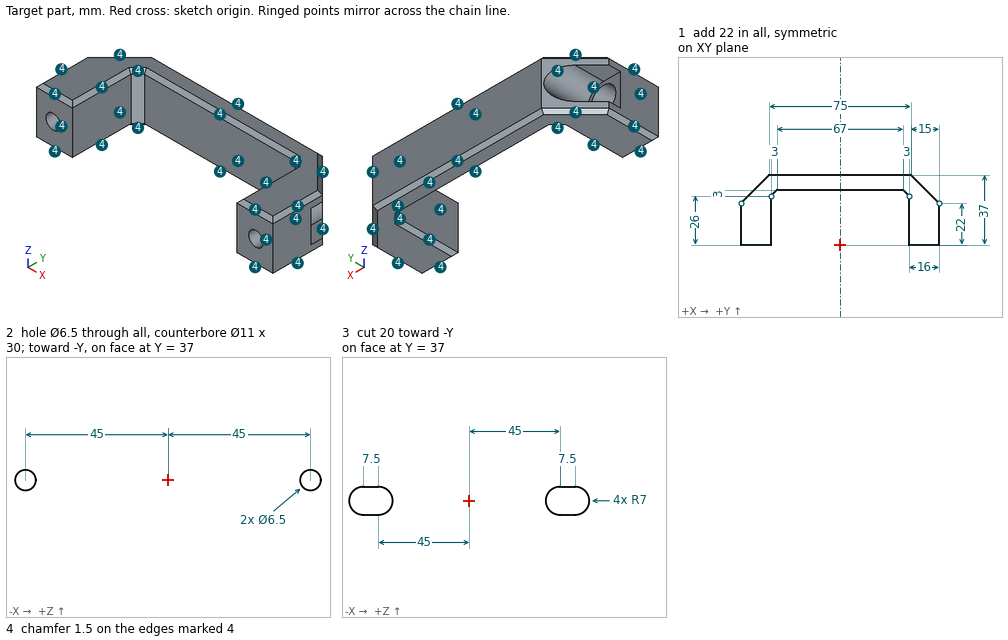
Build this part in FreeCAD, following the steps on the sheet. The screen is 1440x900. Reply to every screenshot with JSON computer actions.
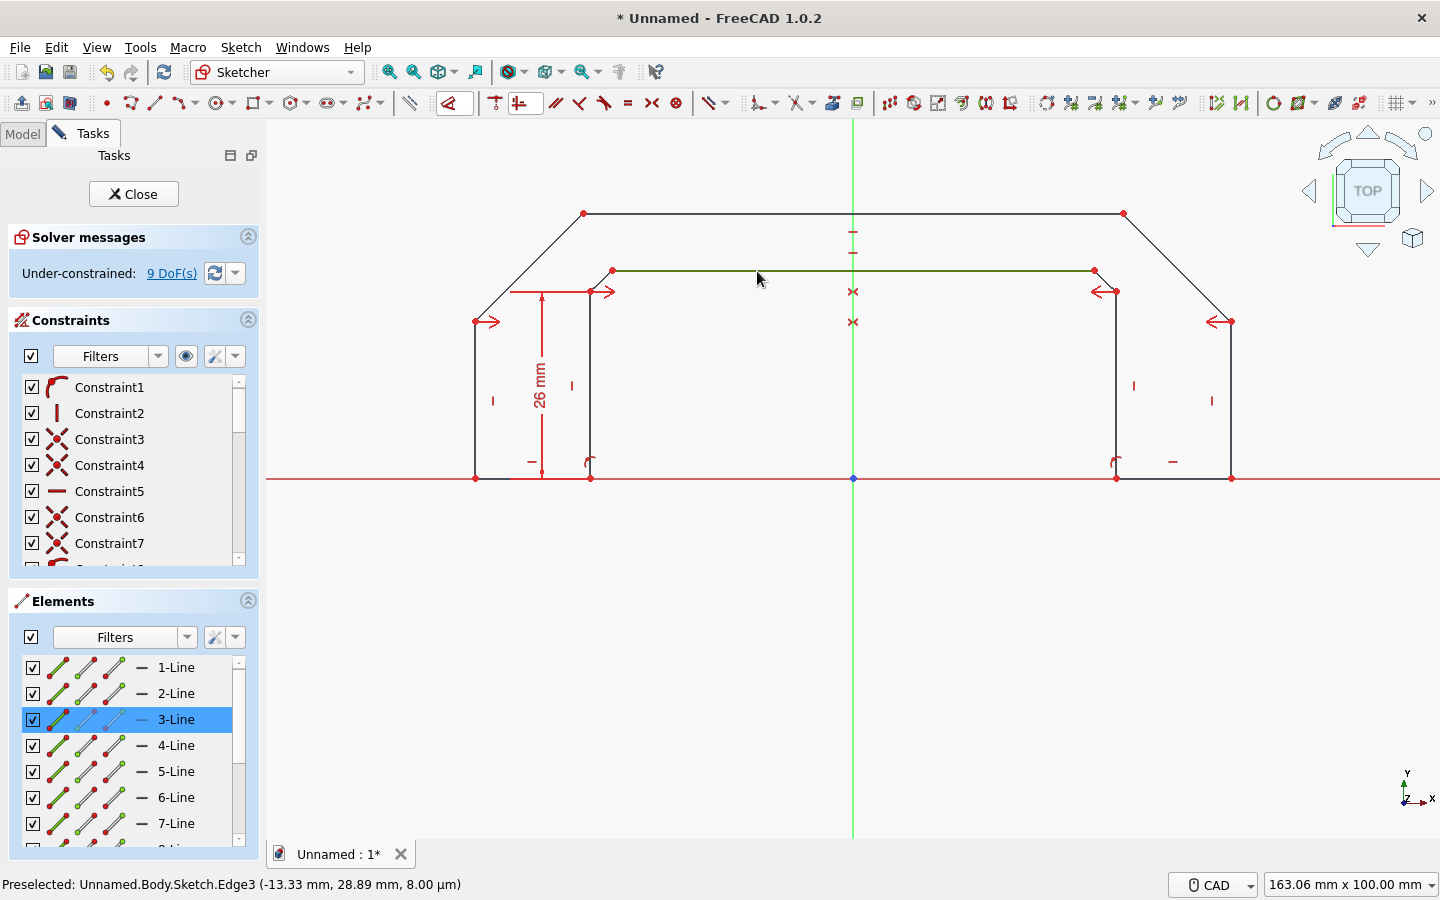
{"action": "left_click", "coordinate": [468, 104]}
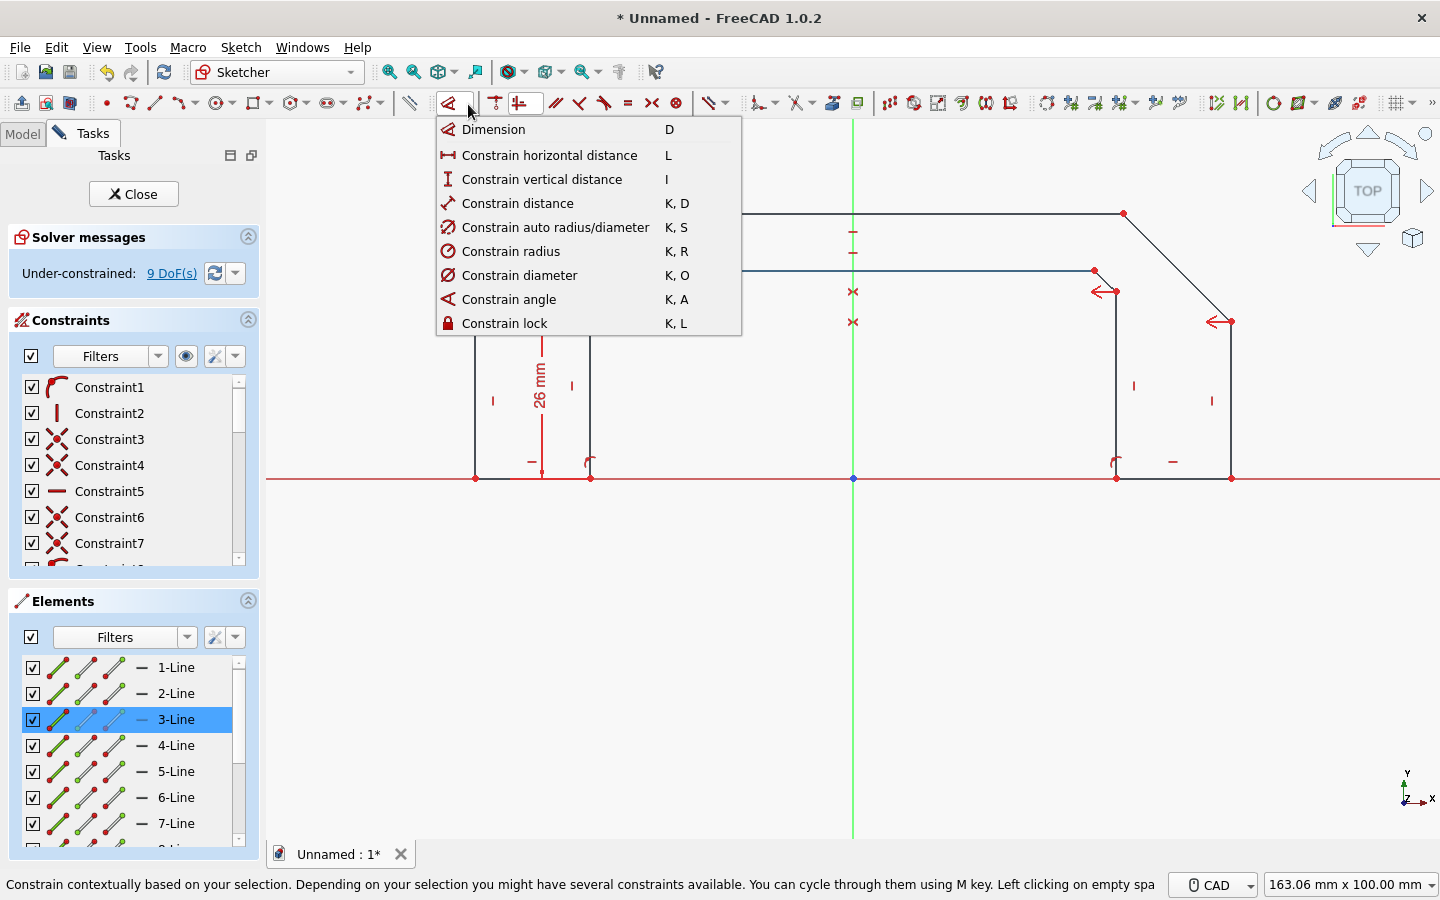
{"action": "left_click", "coordinate": [589, 155]}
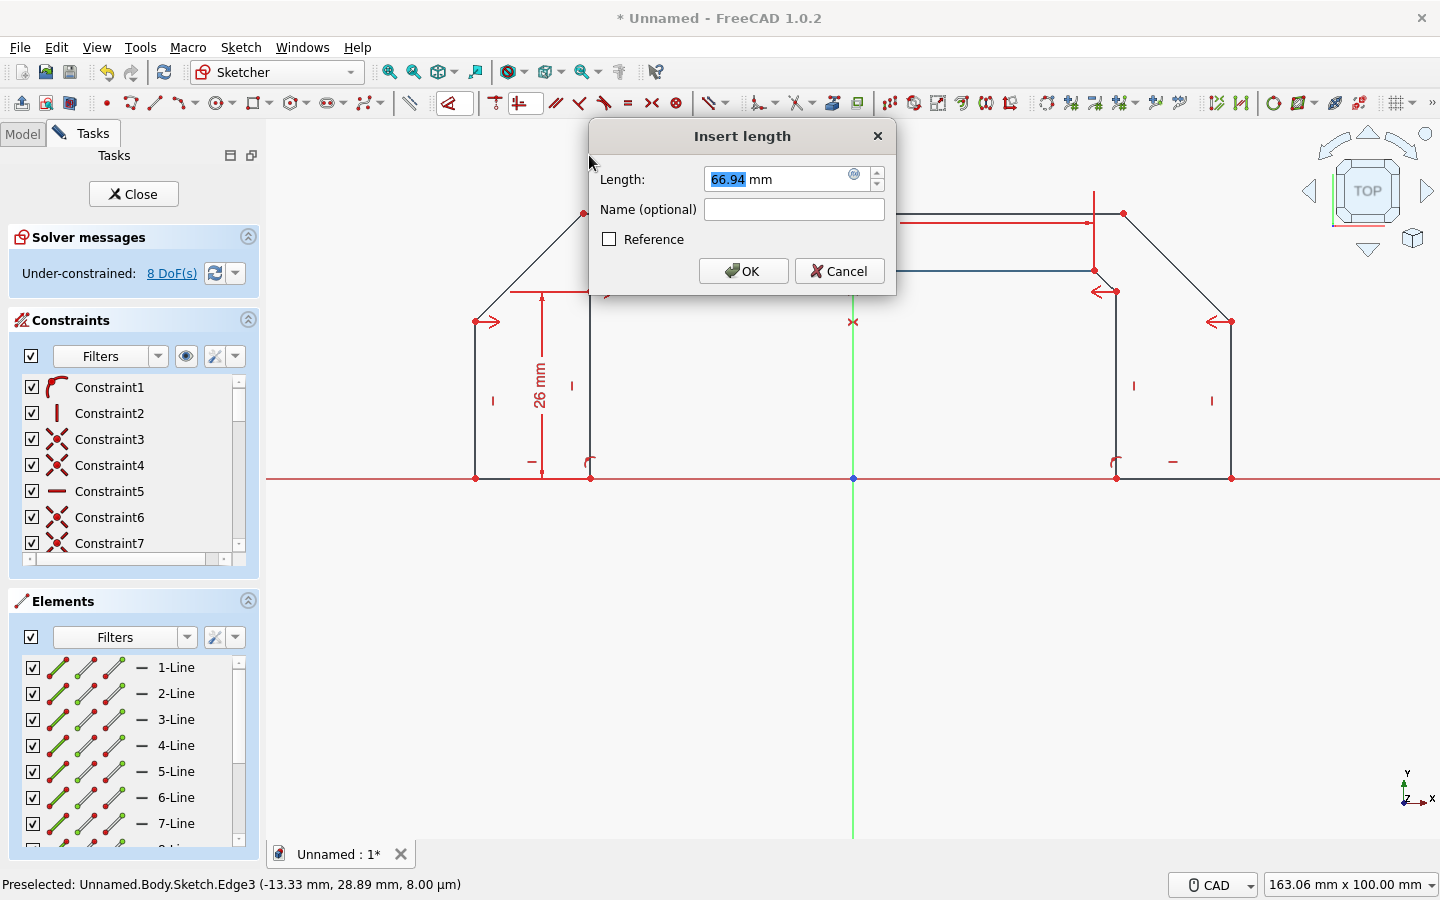
{"action": "type", "text": "67"}
{"action": "key", "text": "Return"}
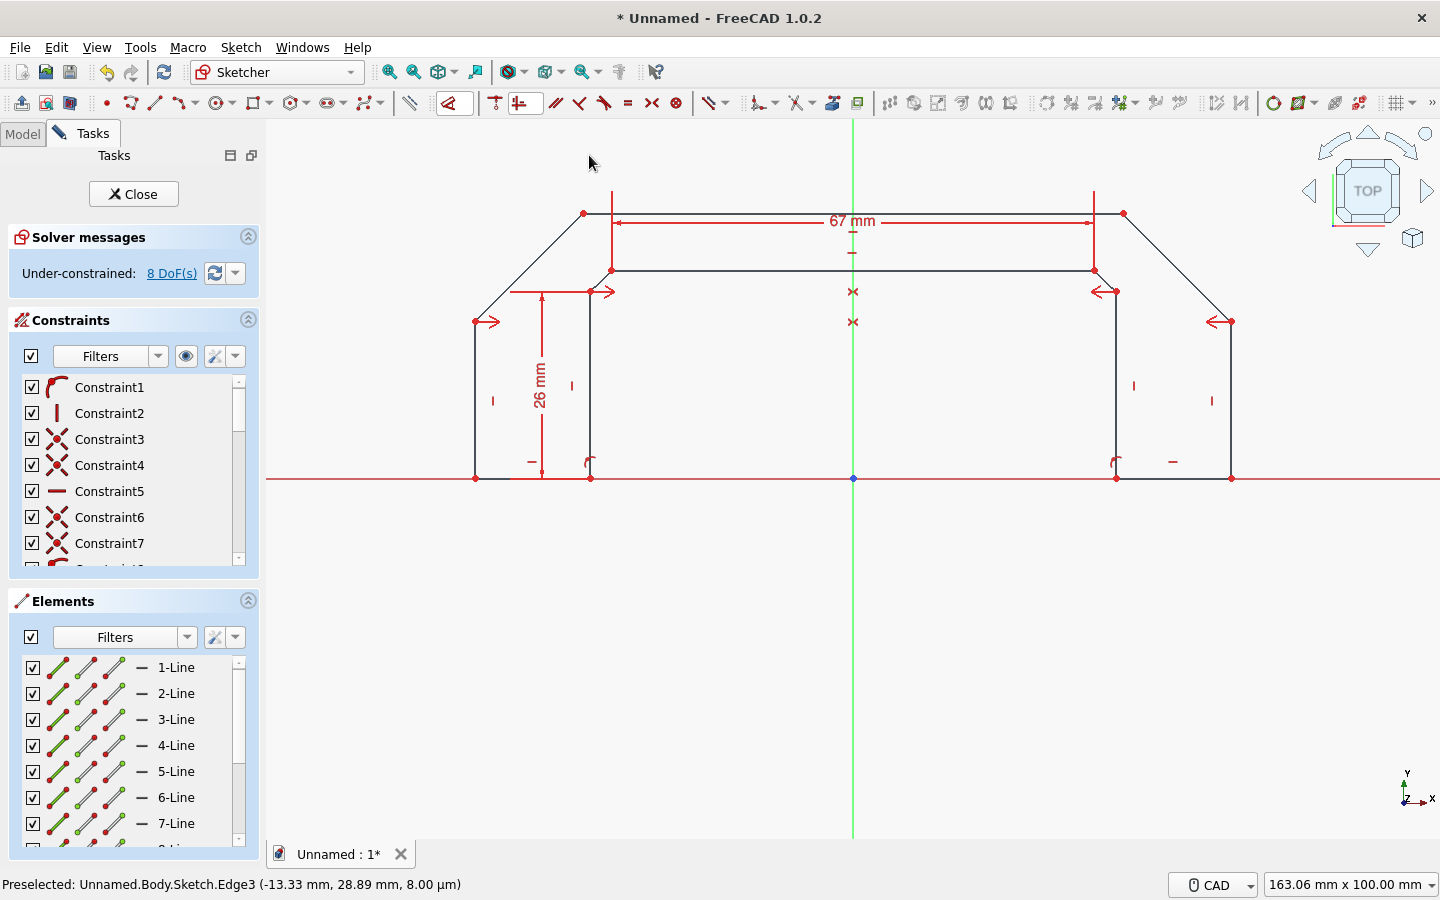
{"action": "left_click", "coordinate": [1150, 479]}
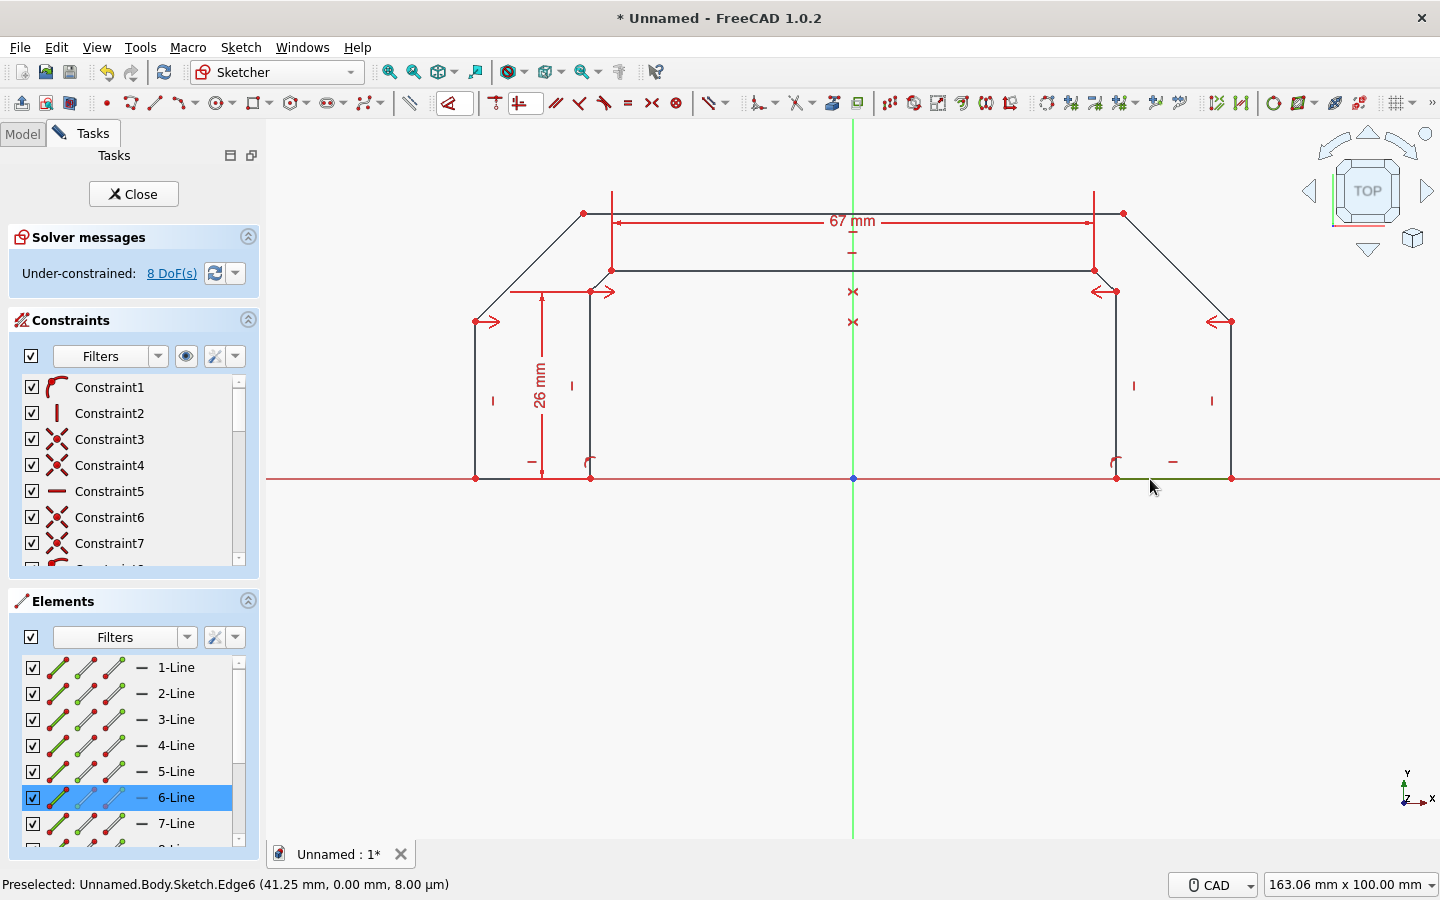
{"action": "left_click", "coordinate": [468, 104]}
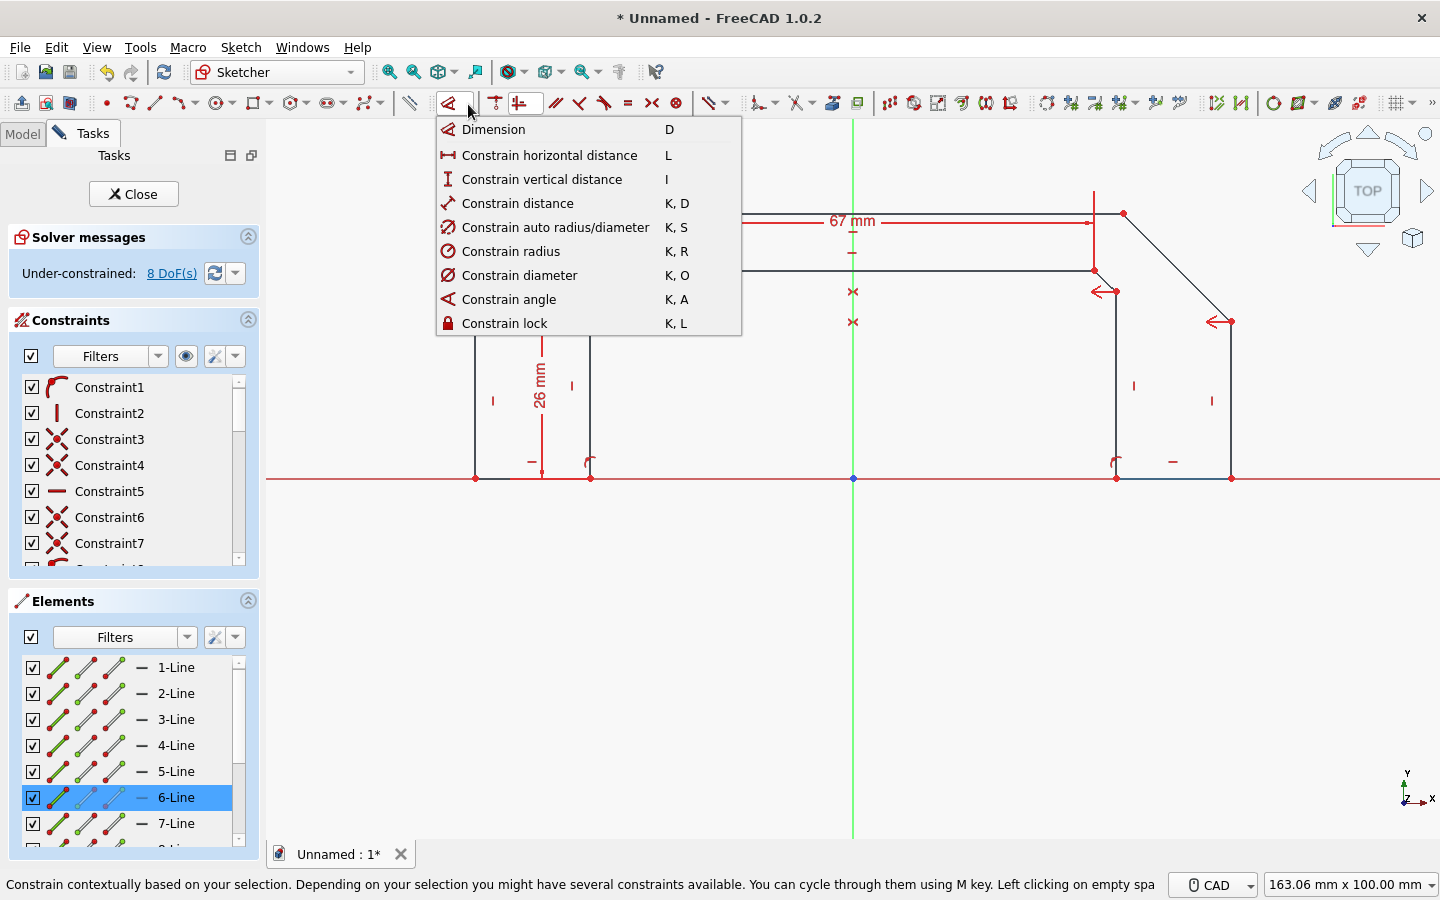
{"action": "left_click", "coordinate": [589, 155]}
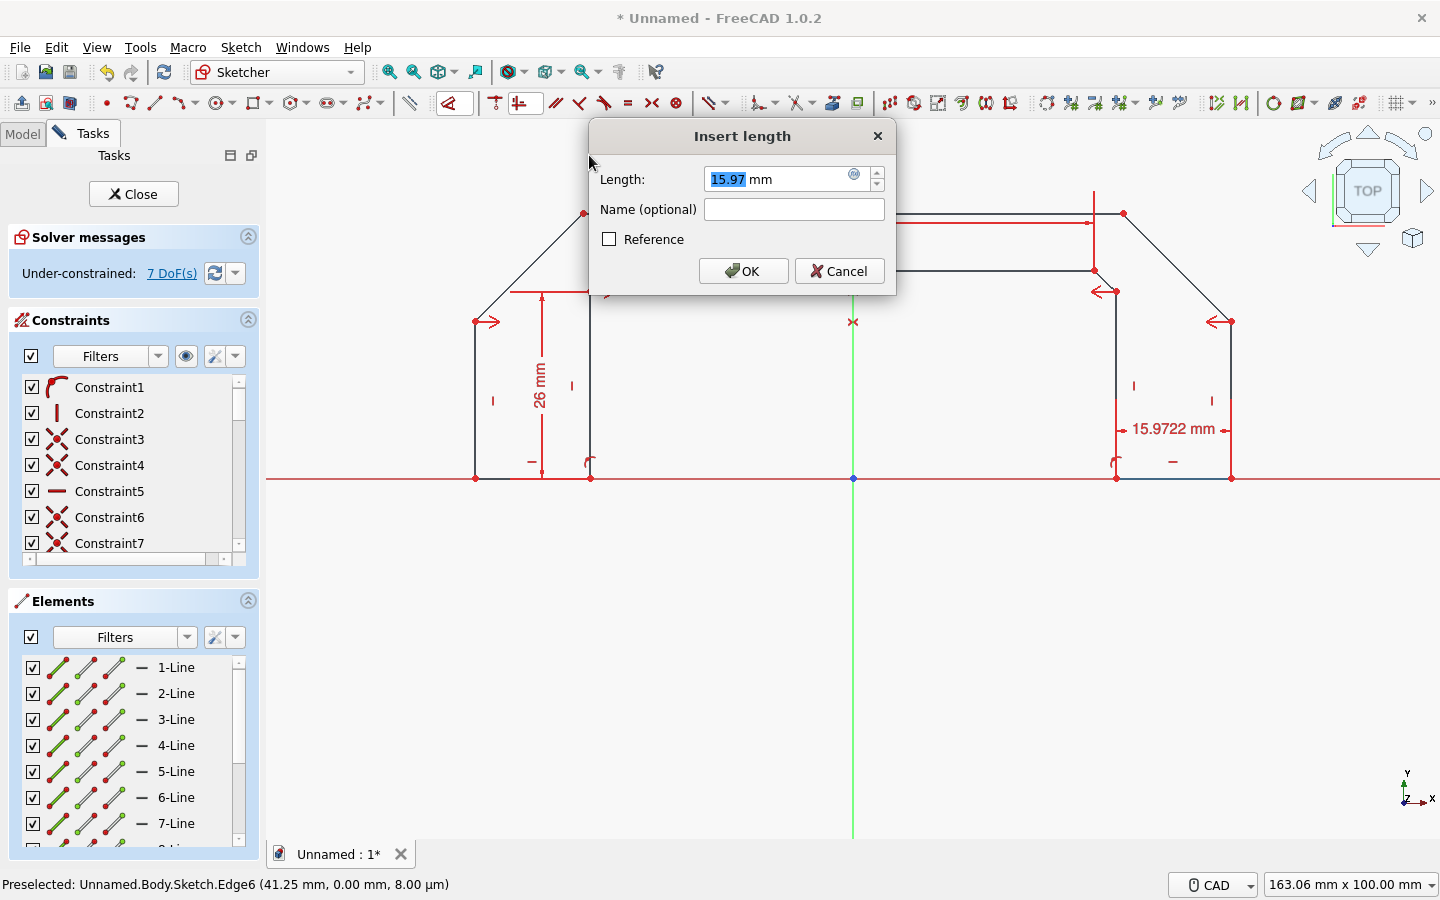
{"action": "type", "text": "16"}
{"action": "key", "text": "Return"}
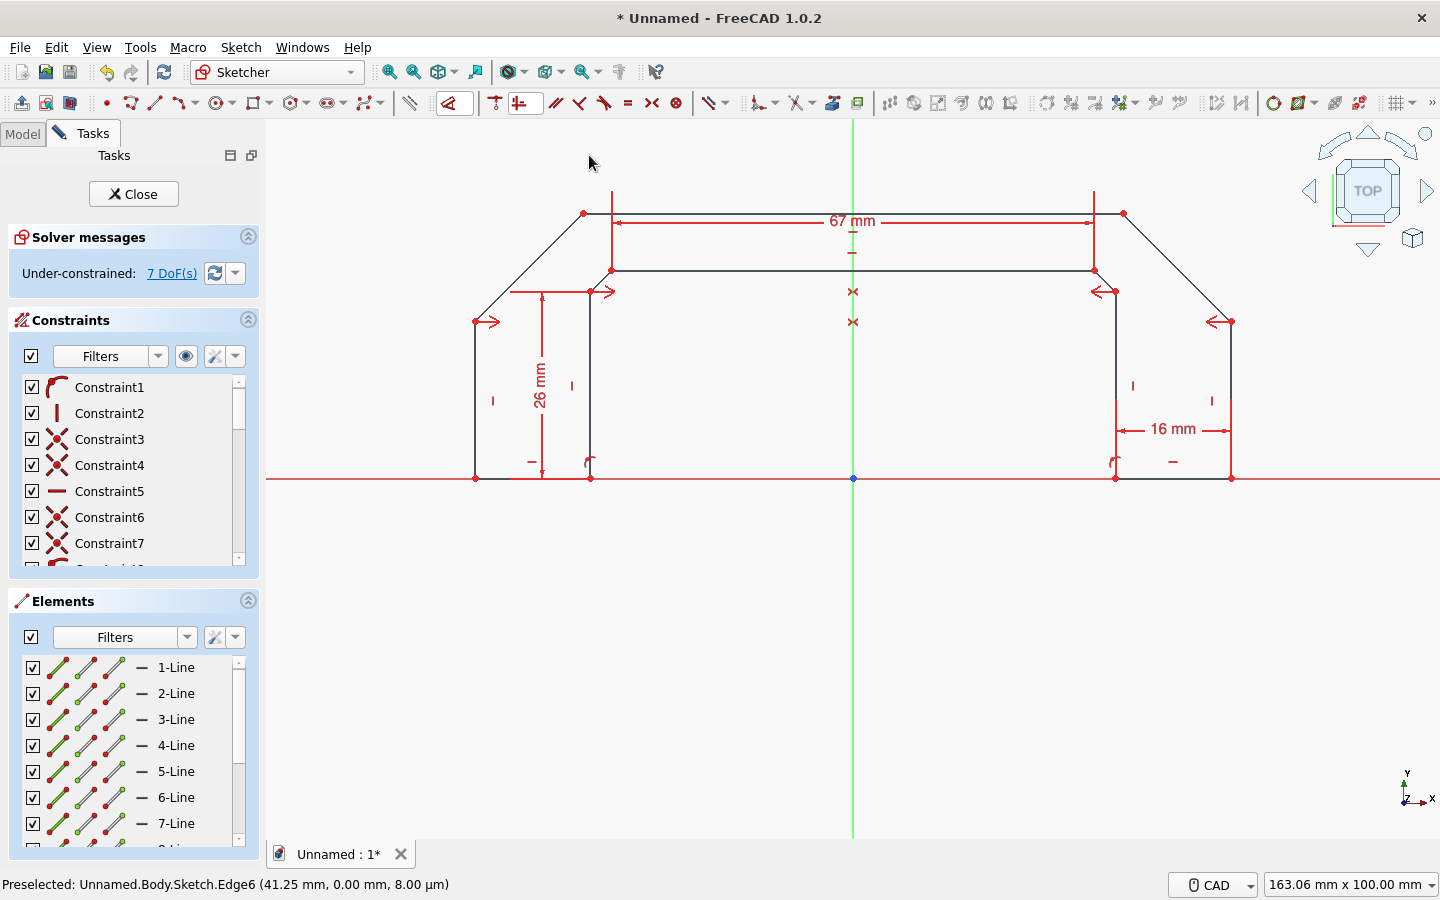
{"action": "left_click", "coordinate": [1231, 432]}